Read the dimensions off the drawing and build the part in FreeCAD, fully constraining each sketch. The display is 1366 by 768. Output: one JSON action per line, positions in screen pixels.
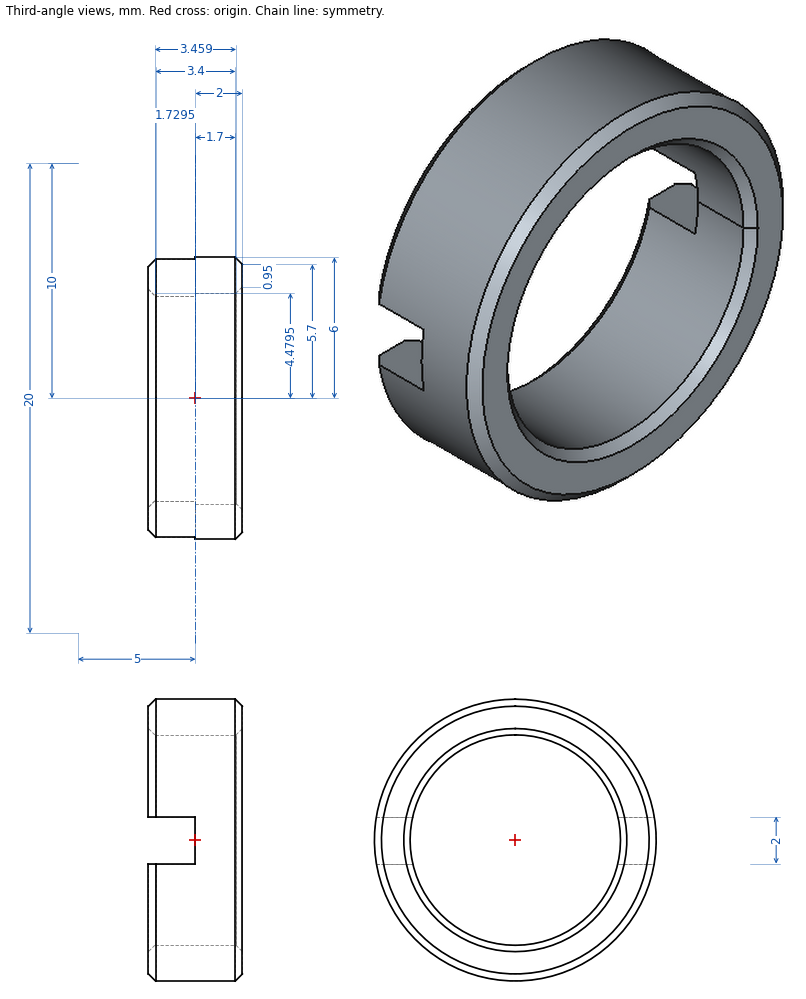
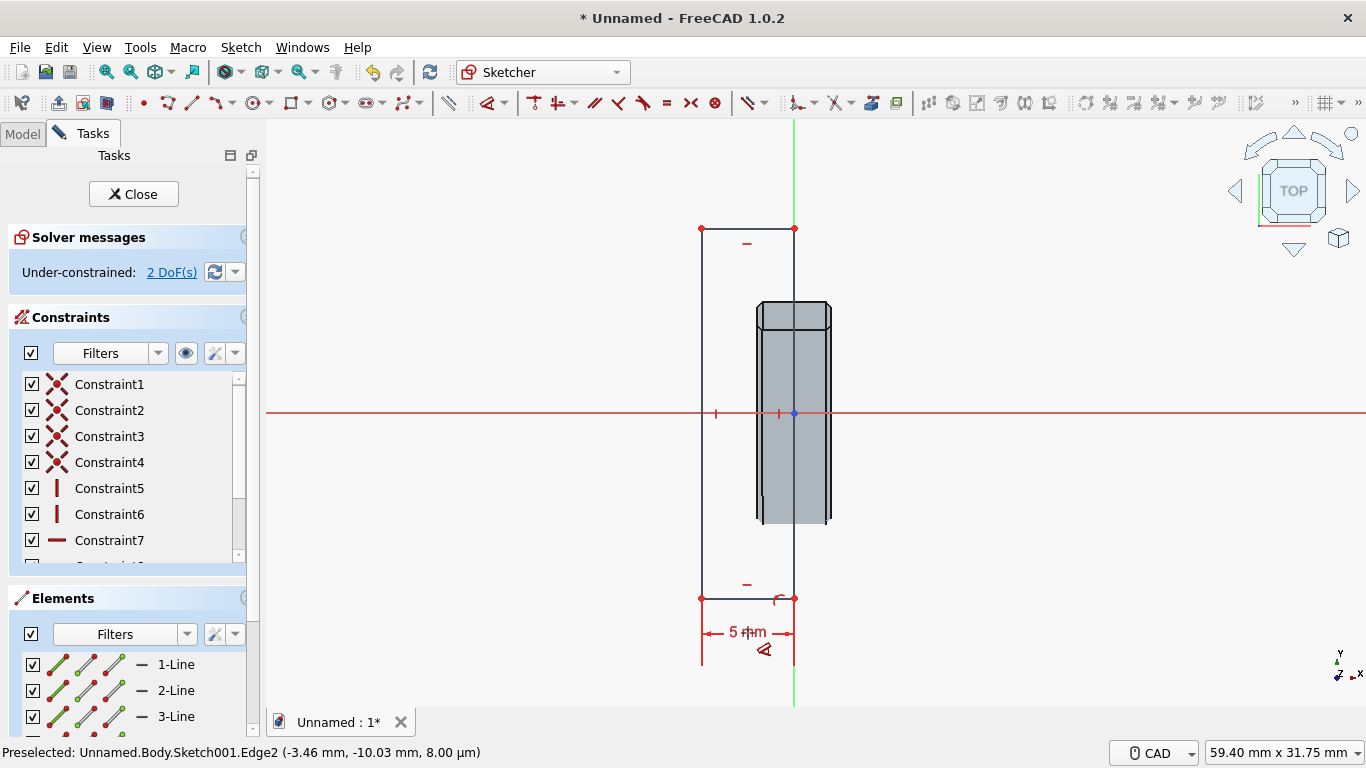
{"action": "left_click", "coordinate": [702, 340]}
{"action": "left_click", "coordinate": [668, 329]}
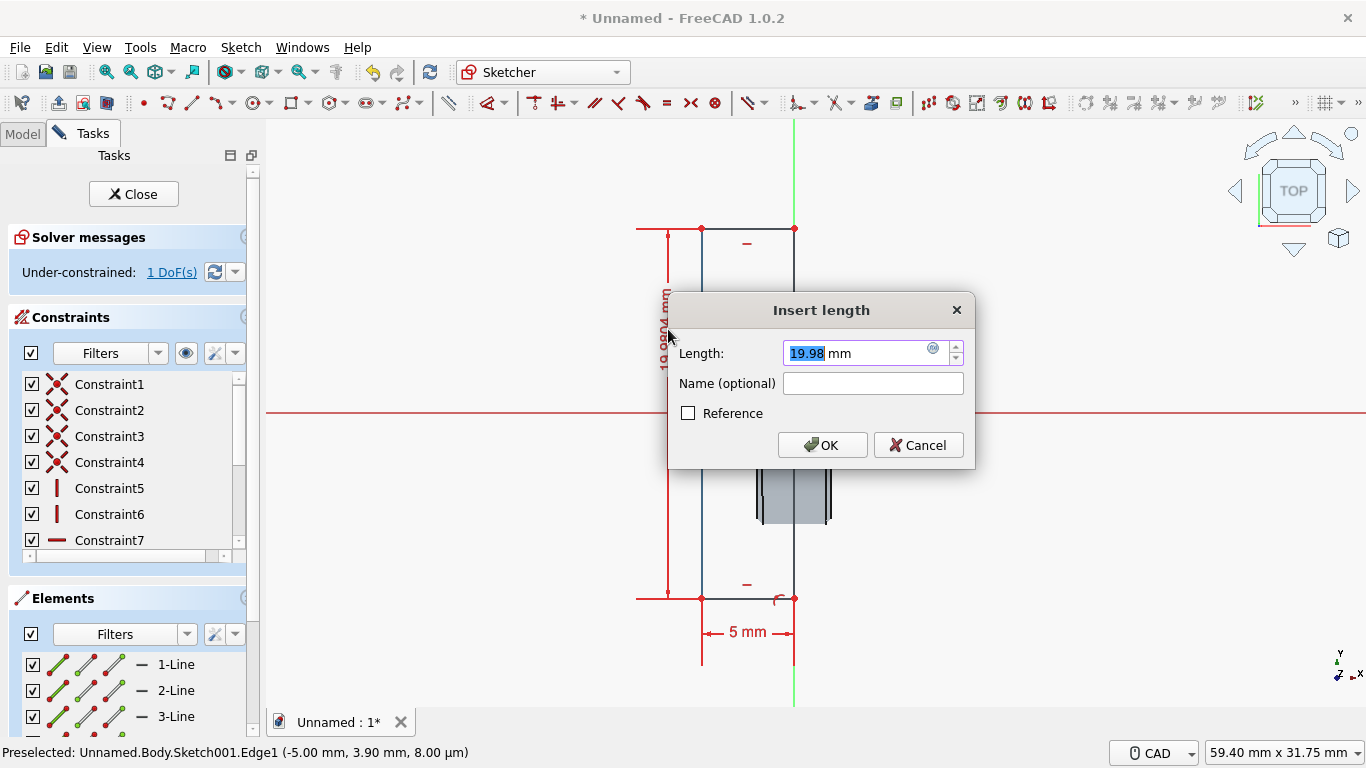
{"action": "type", "text": "20"}
{"action": "key", "text": "Return"}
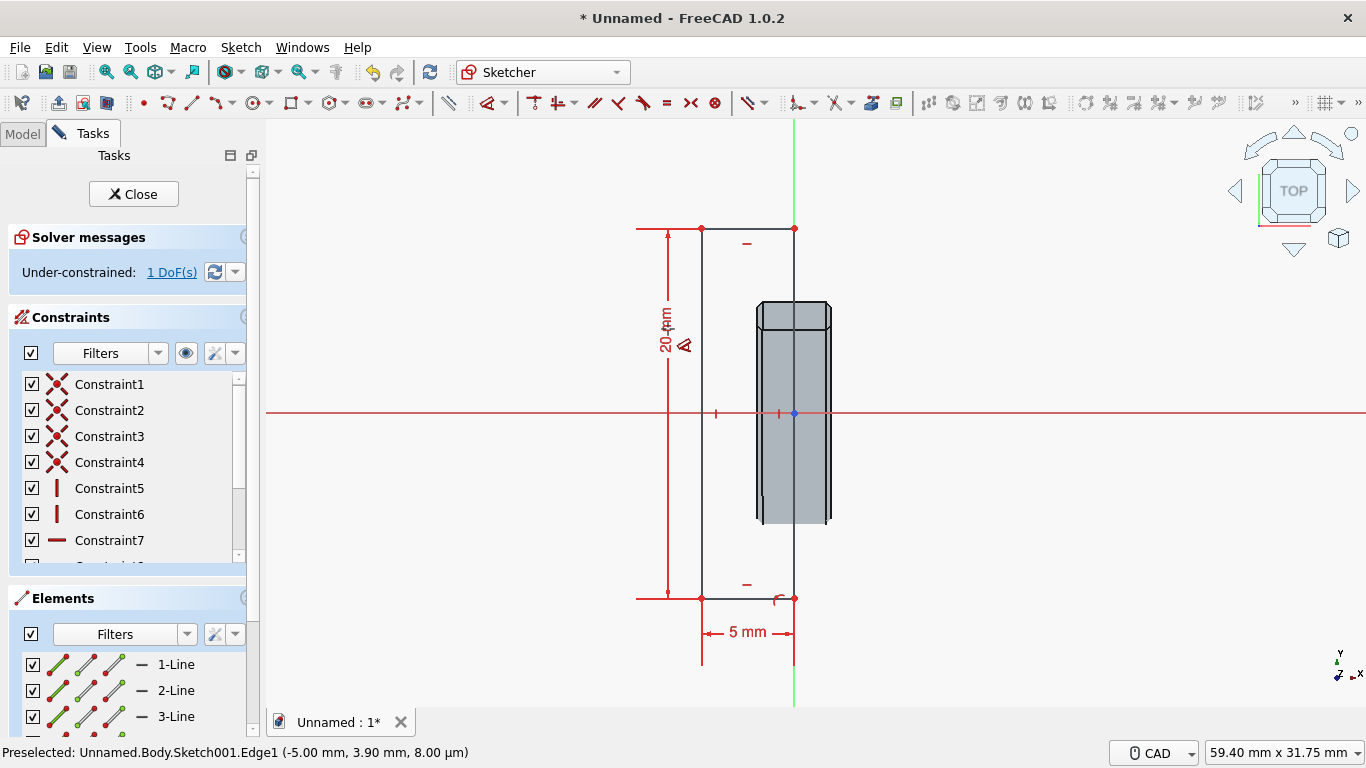
{"action": "left_click", "coordinate": [702, 229]}
{"action": "left_click", "coordinate": [828, 321]}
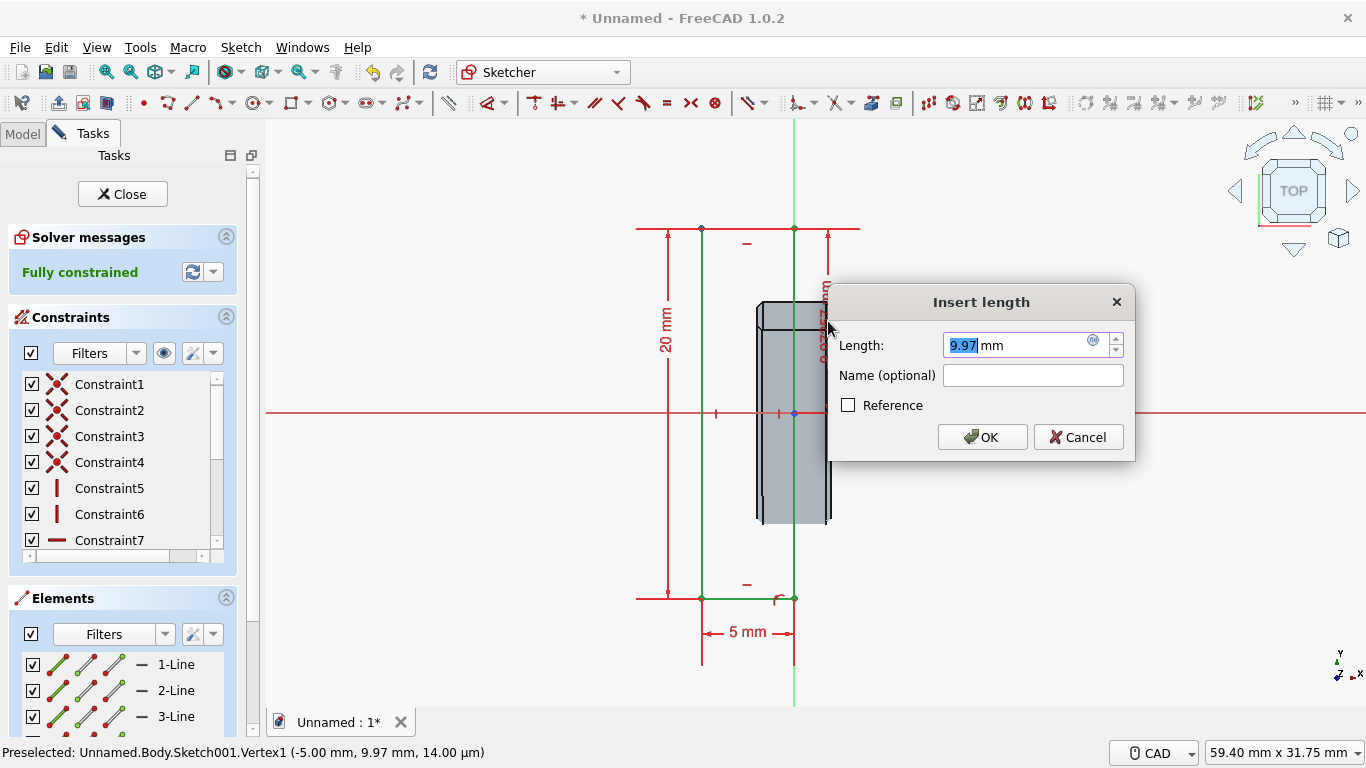
{"action": "type", "text": "10"}
{"action": "key", "text": "Return"}
{"action": "key", "text": "Escape"}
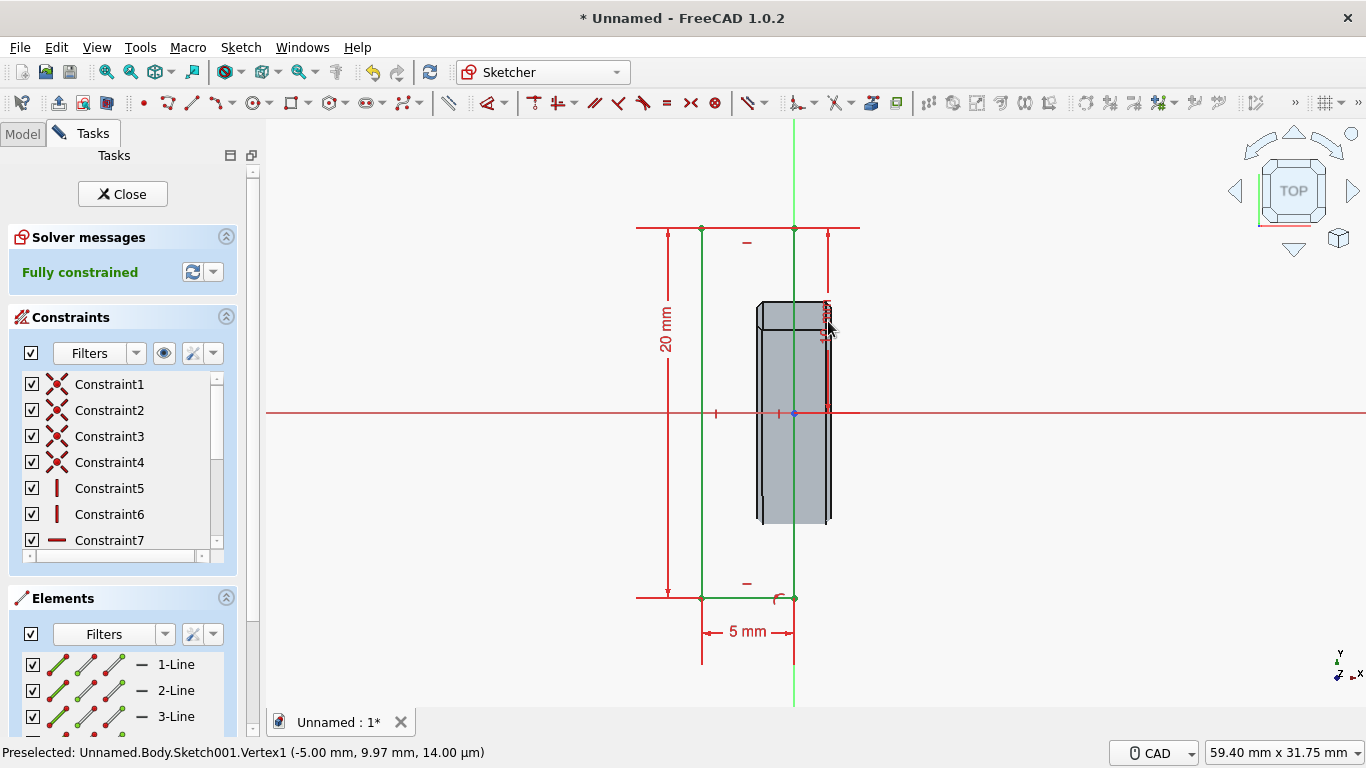
{"action": "left_click", "coordinate": [123, 194]}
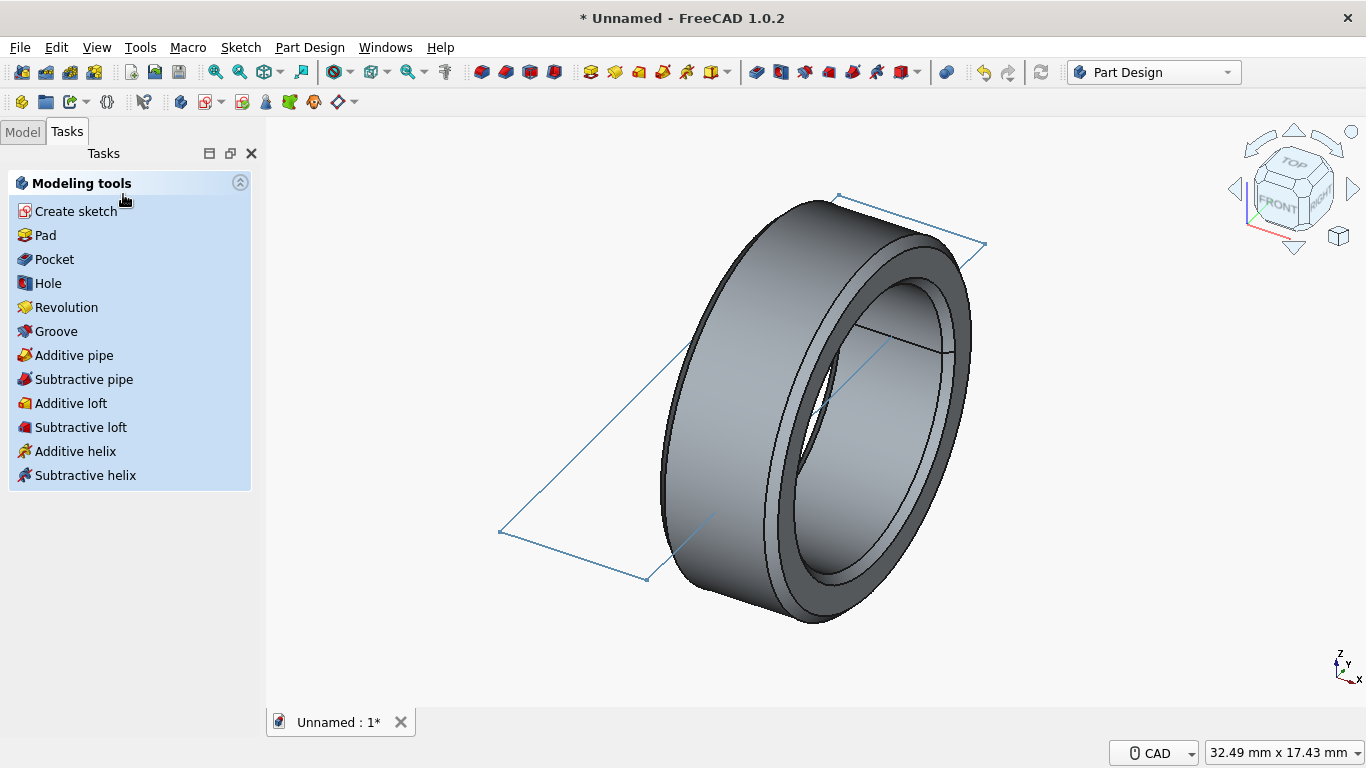
{"action": "left_click", "coordinate": [758, 72]}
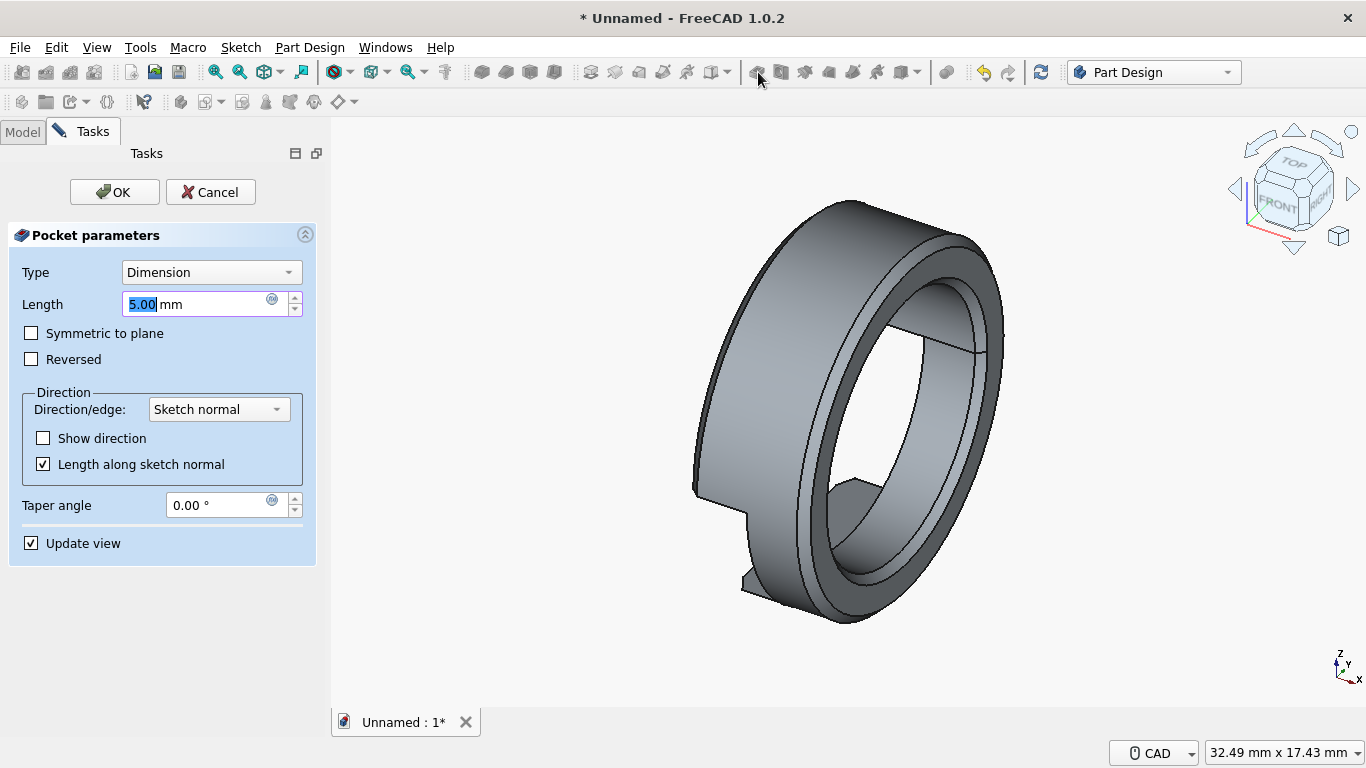
{"action": "type", "text": "2"}
{"action": "key", "text": "Tab"}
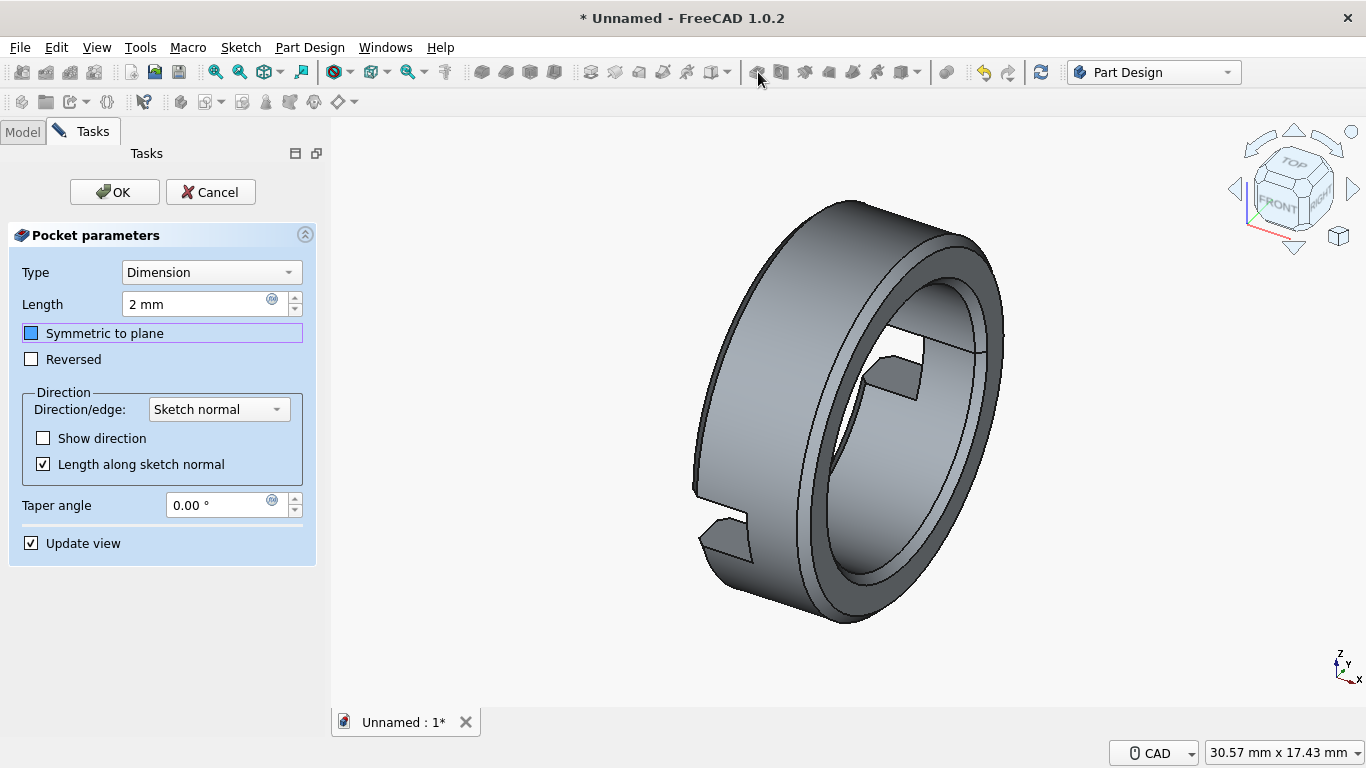
{"action": "left_click", "coordinate": [30, 333]}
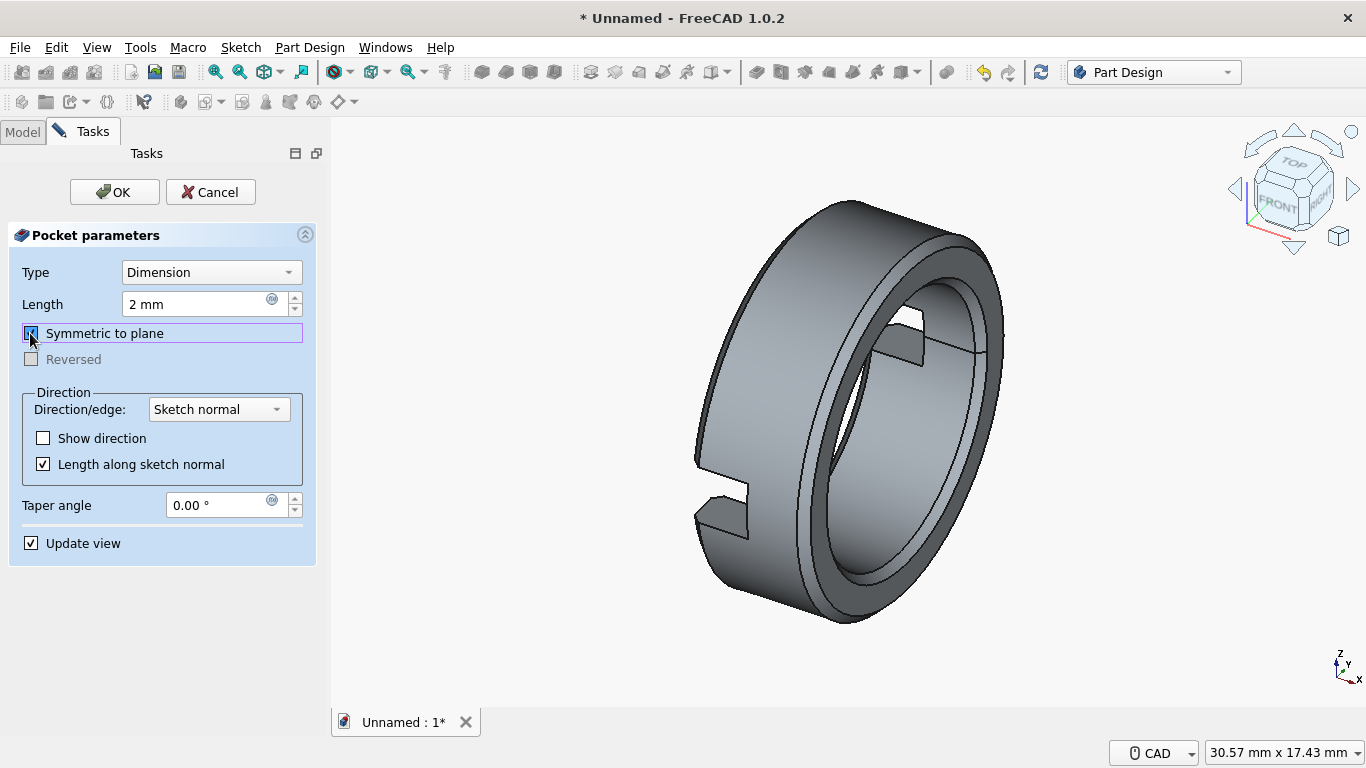
{"action": "left_click", "coordinate": [115, 192]}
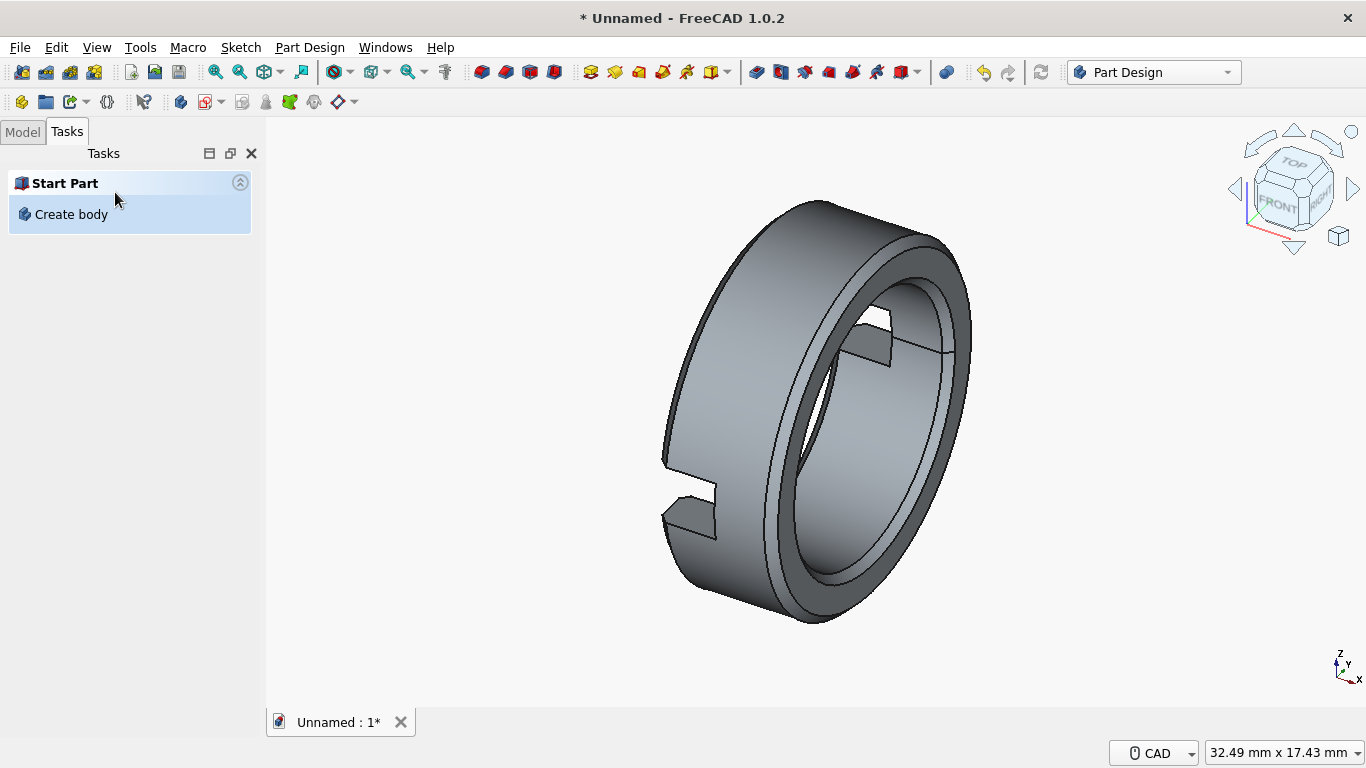
{"action": "key", "text": "0"}